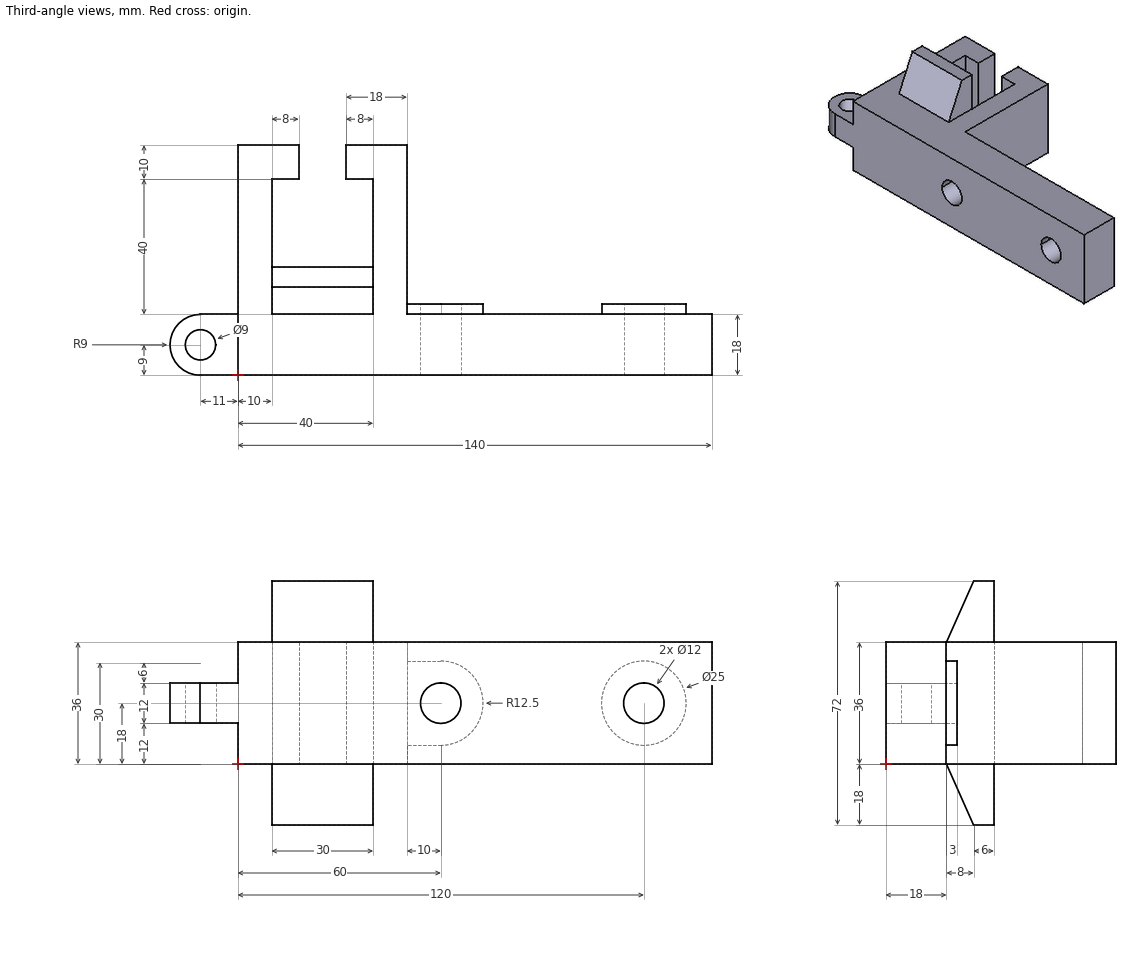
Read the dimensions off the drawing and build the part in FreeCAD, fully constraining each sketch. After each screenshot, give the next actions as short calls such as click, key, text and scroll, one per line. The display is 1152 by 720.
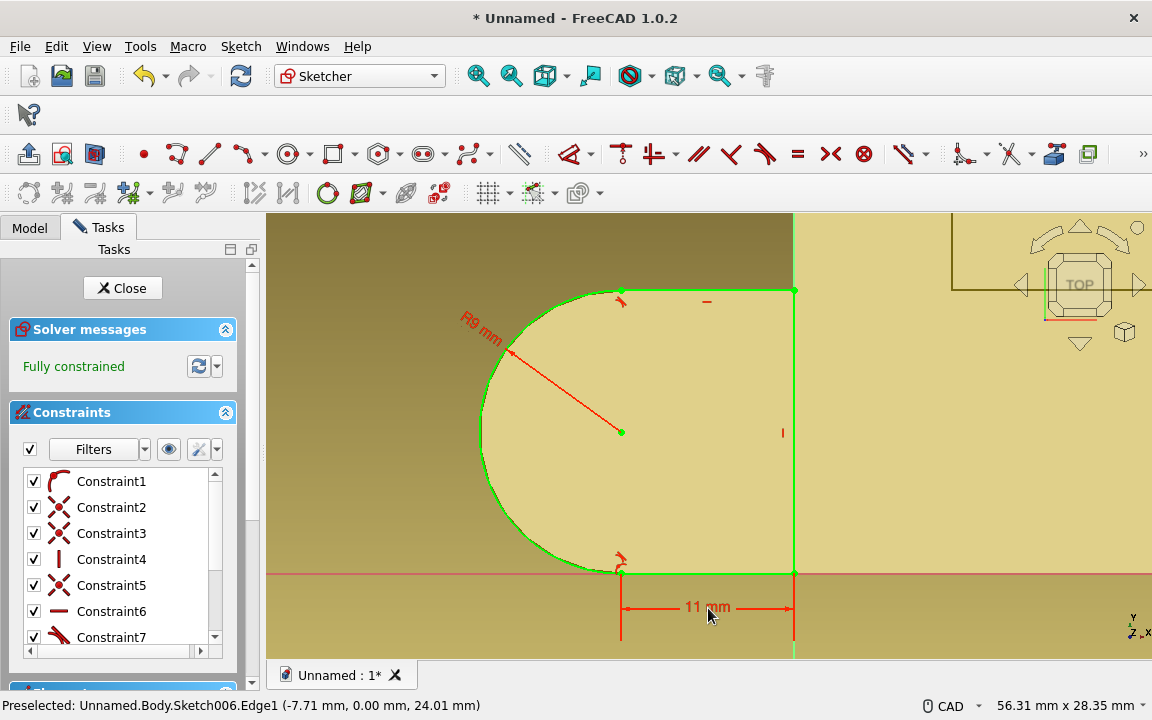
click(123, 288)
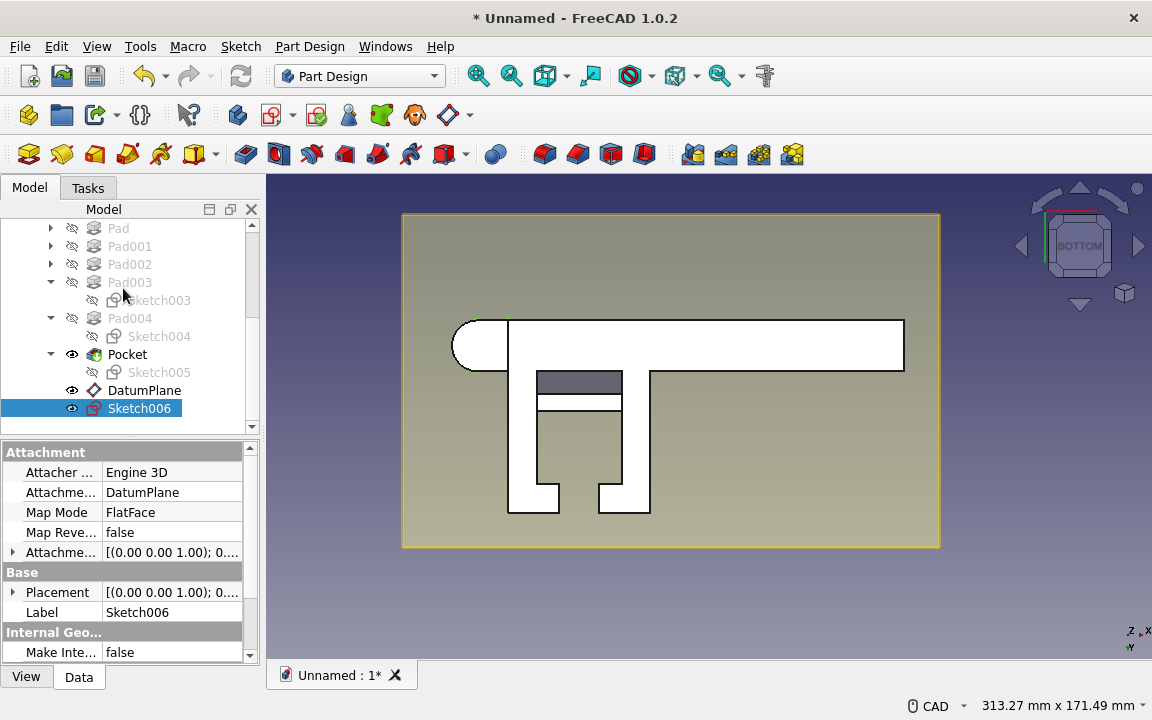
click(246, 154)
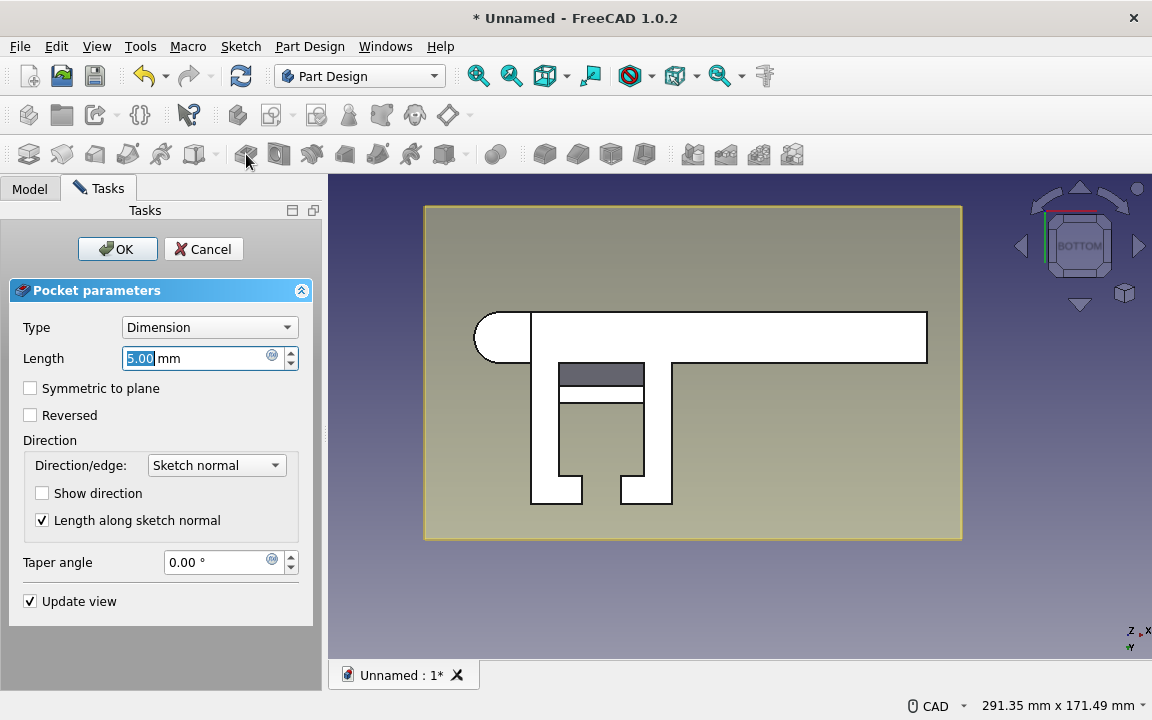
text(6)
key(Tab)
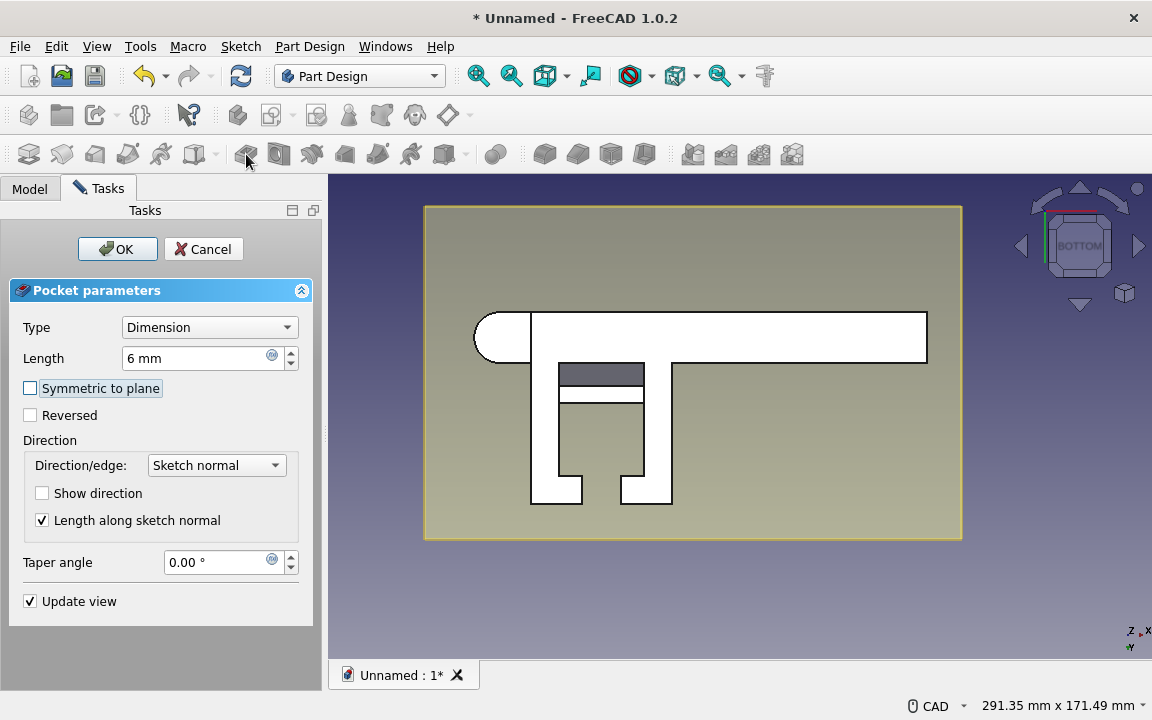
click(31, 415)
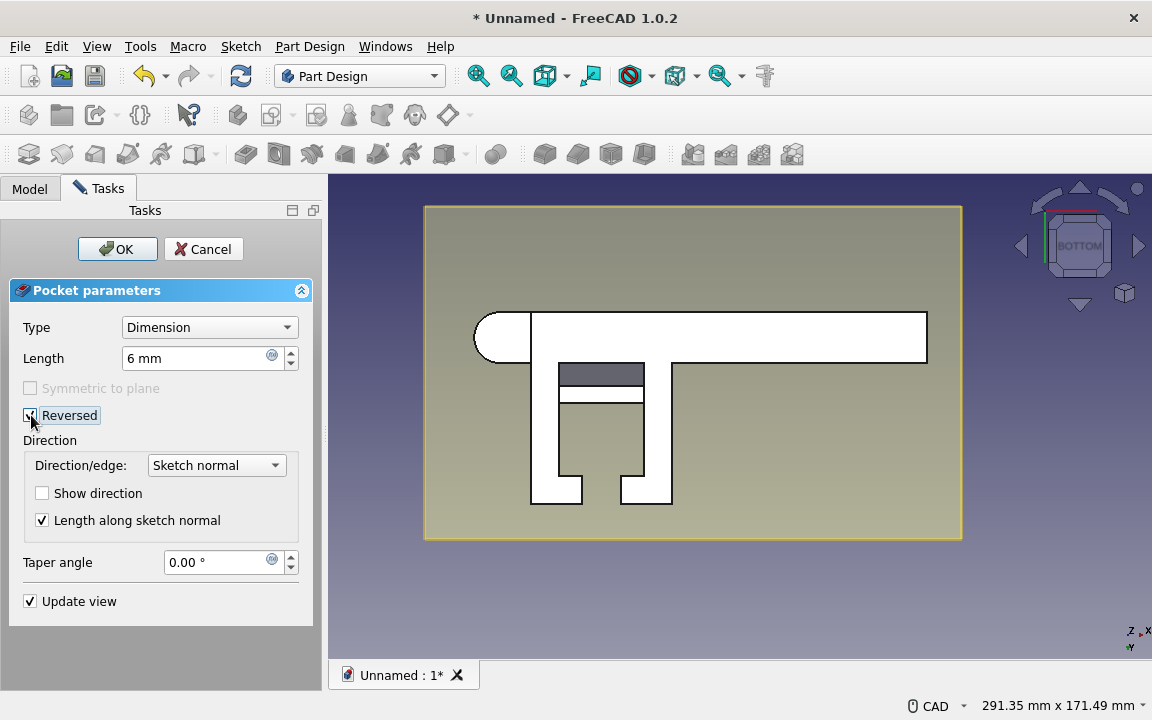
click(118, 249)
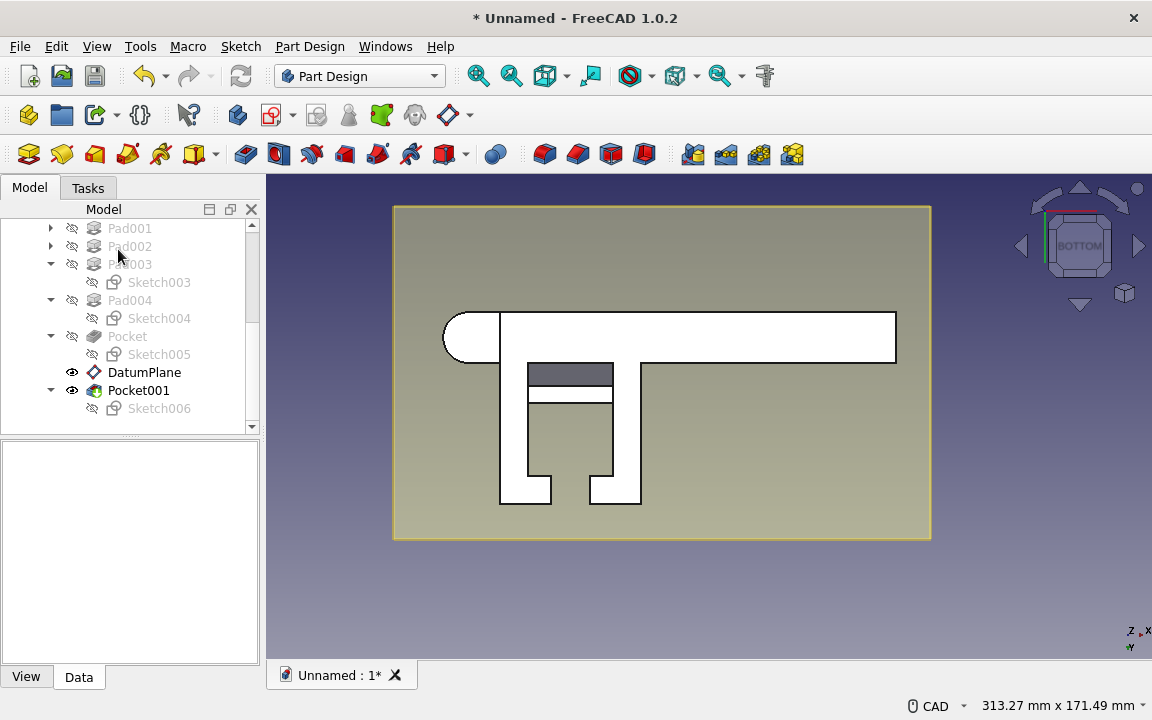
click(117, 372)
key(space)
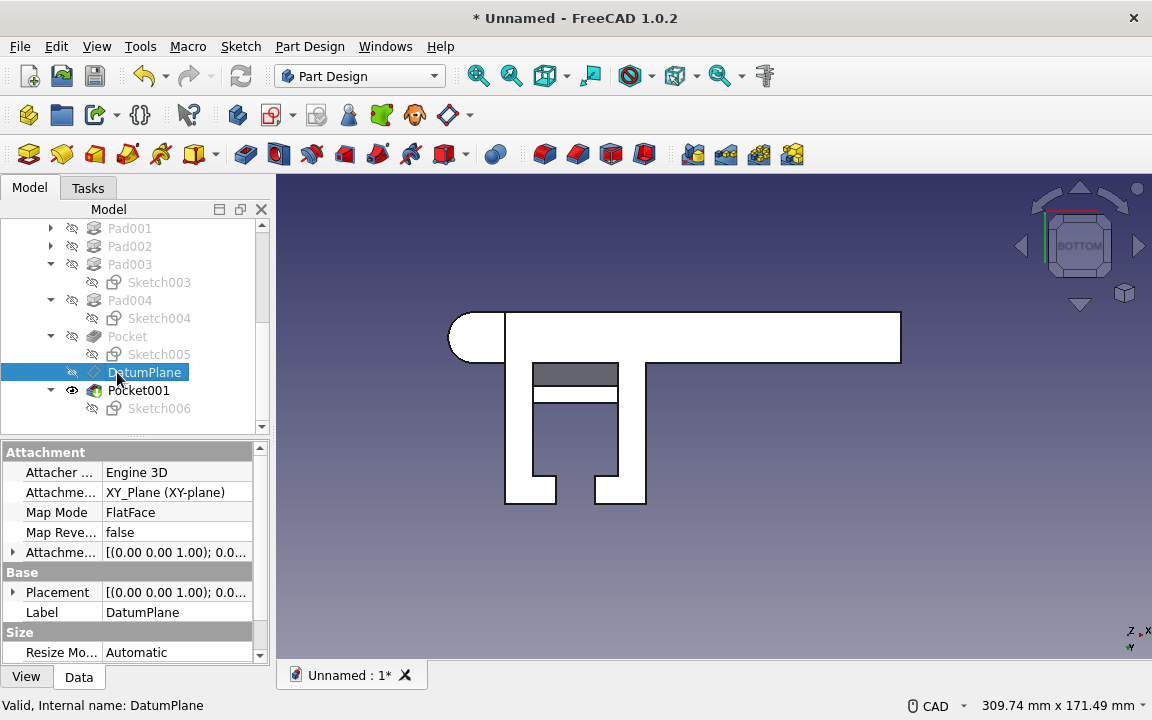
key(0)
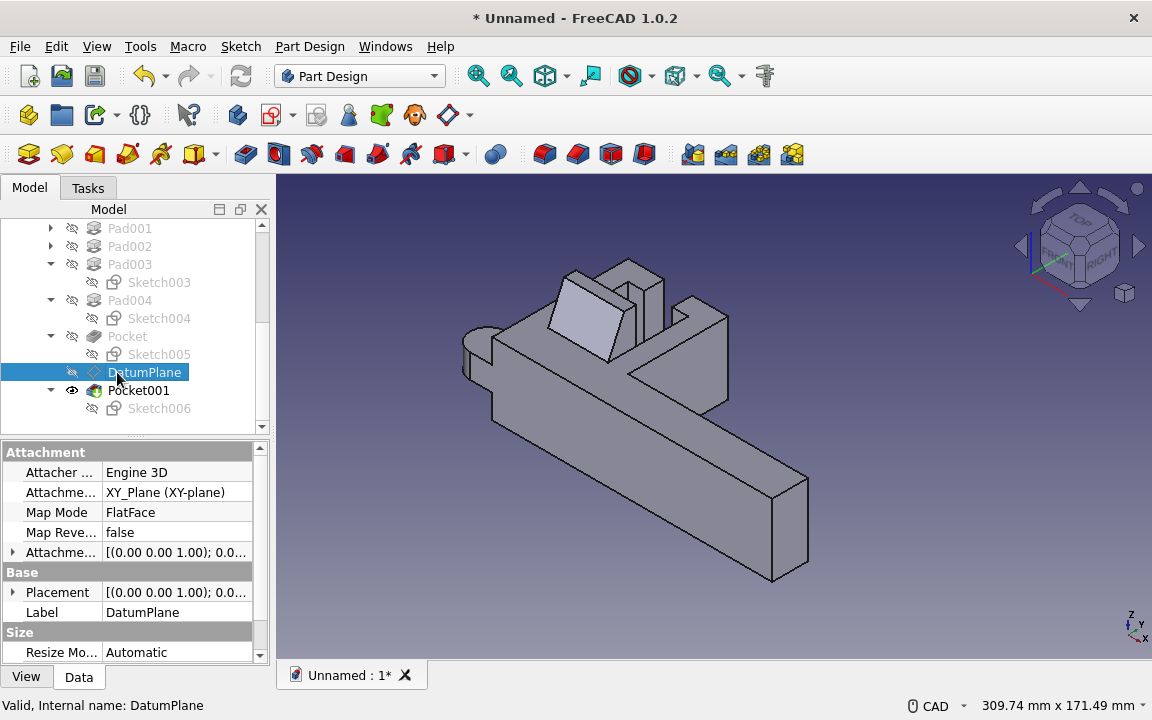
click(484, 339)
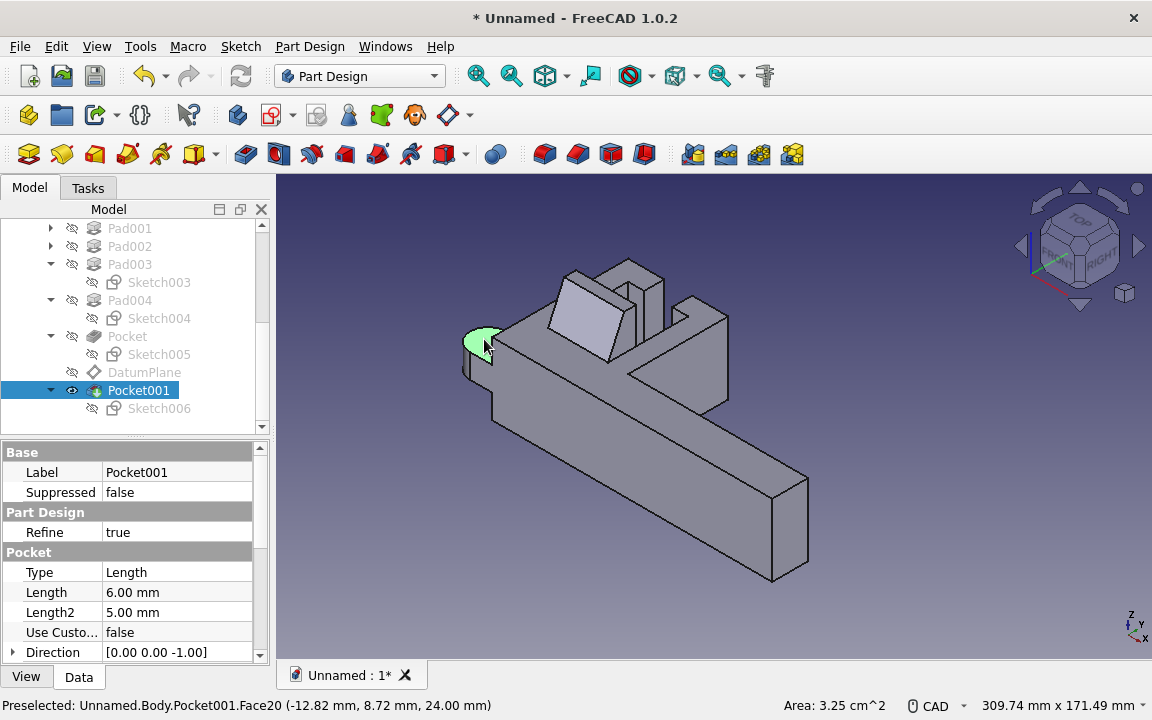
click(270, 116)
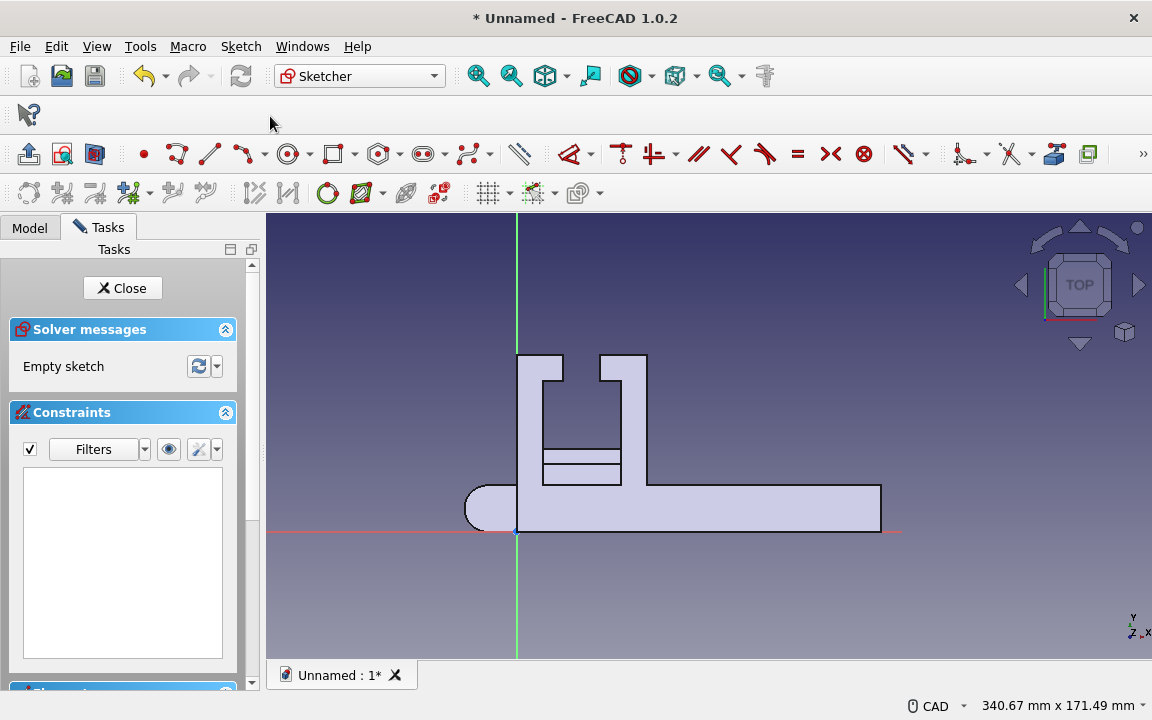
click(95, 154)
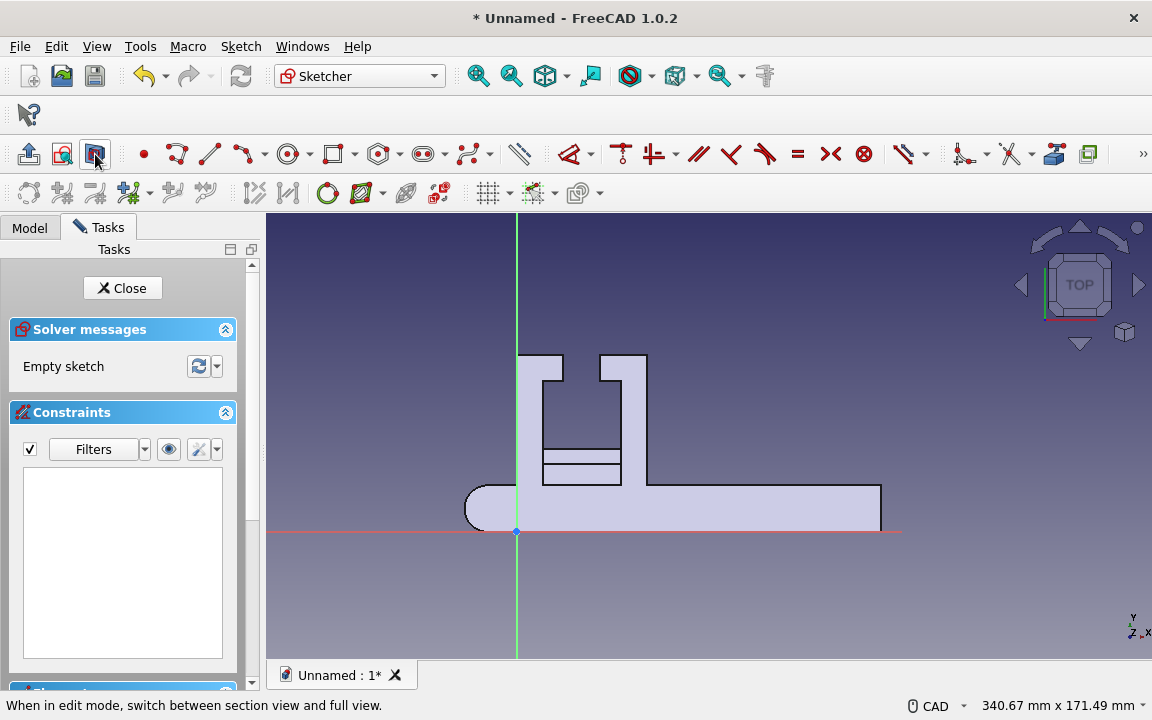
scroll(474, 527, up, 10)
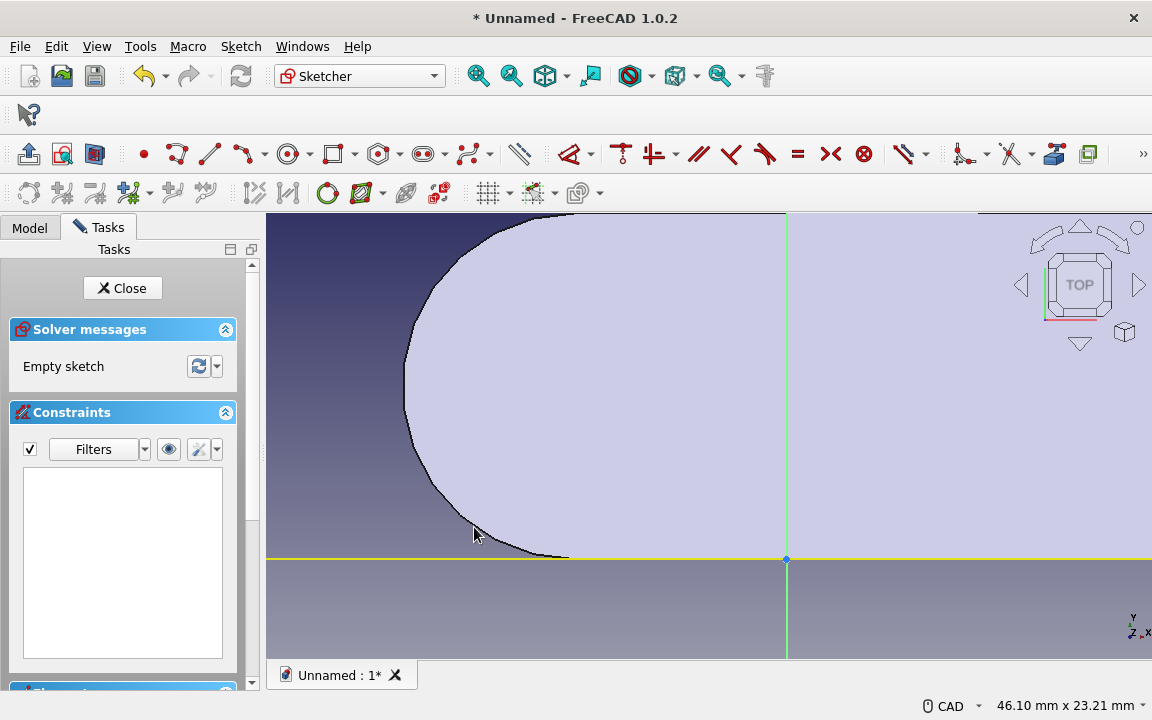
key(g)
key(c)